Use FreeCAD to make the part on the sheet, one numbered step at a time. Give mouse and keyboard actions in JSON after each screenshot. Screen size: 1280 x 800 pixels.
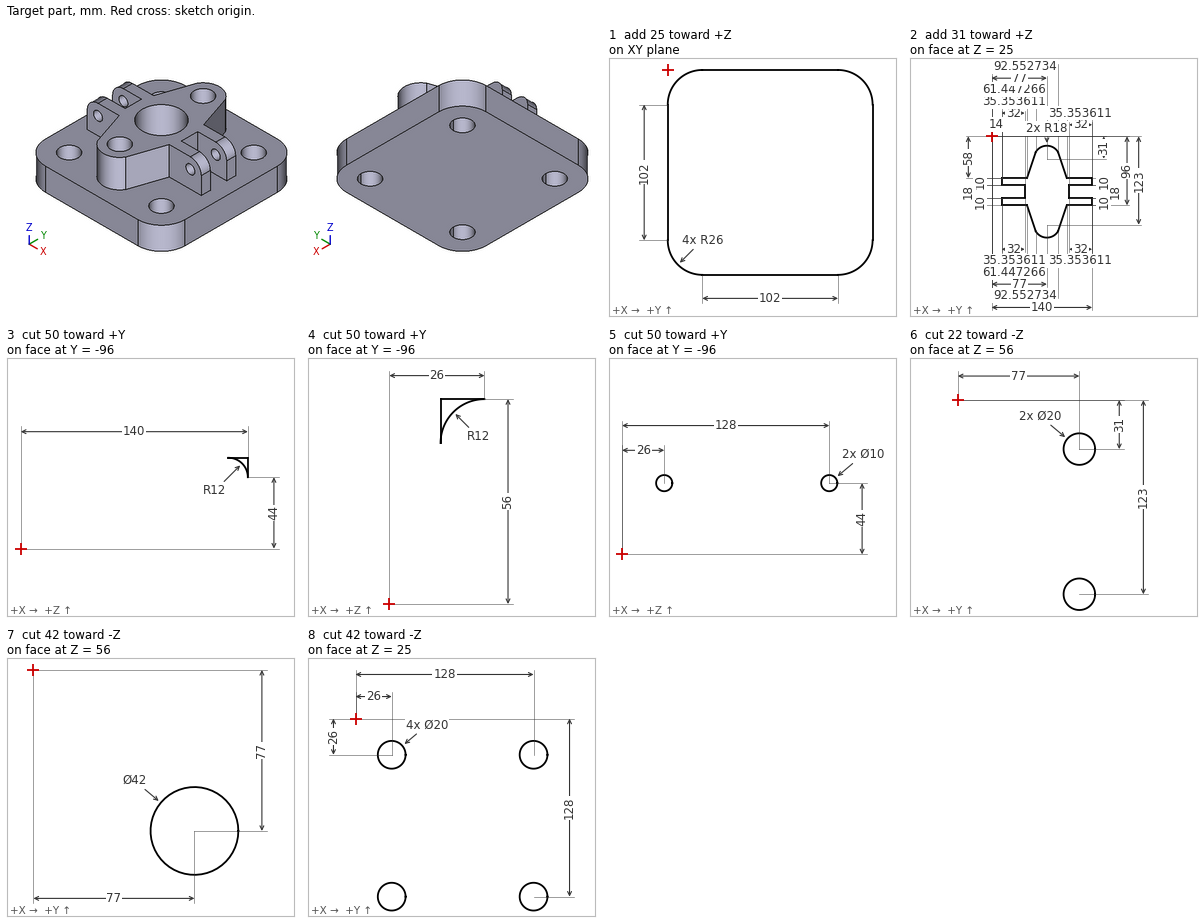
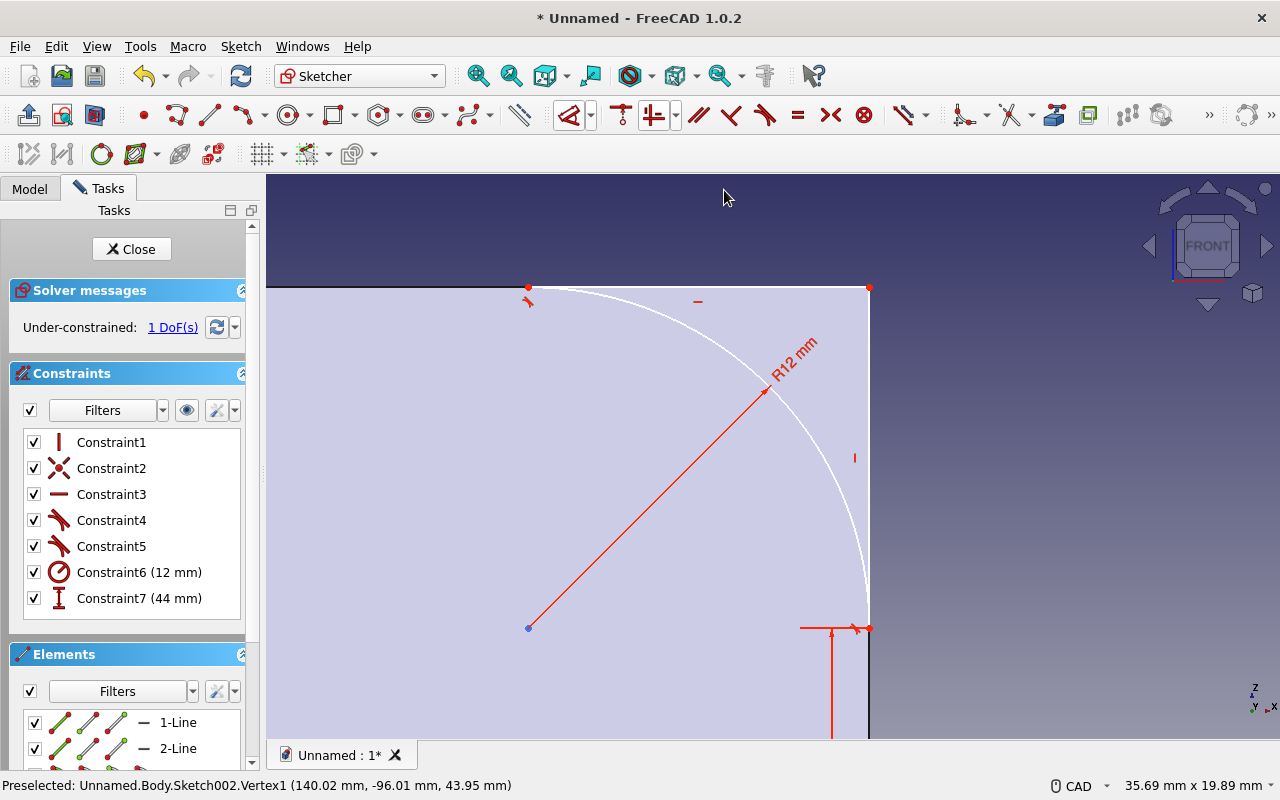
{"action": "left_click", "coordinate": [869, 628]}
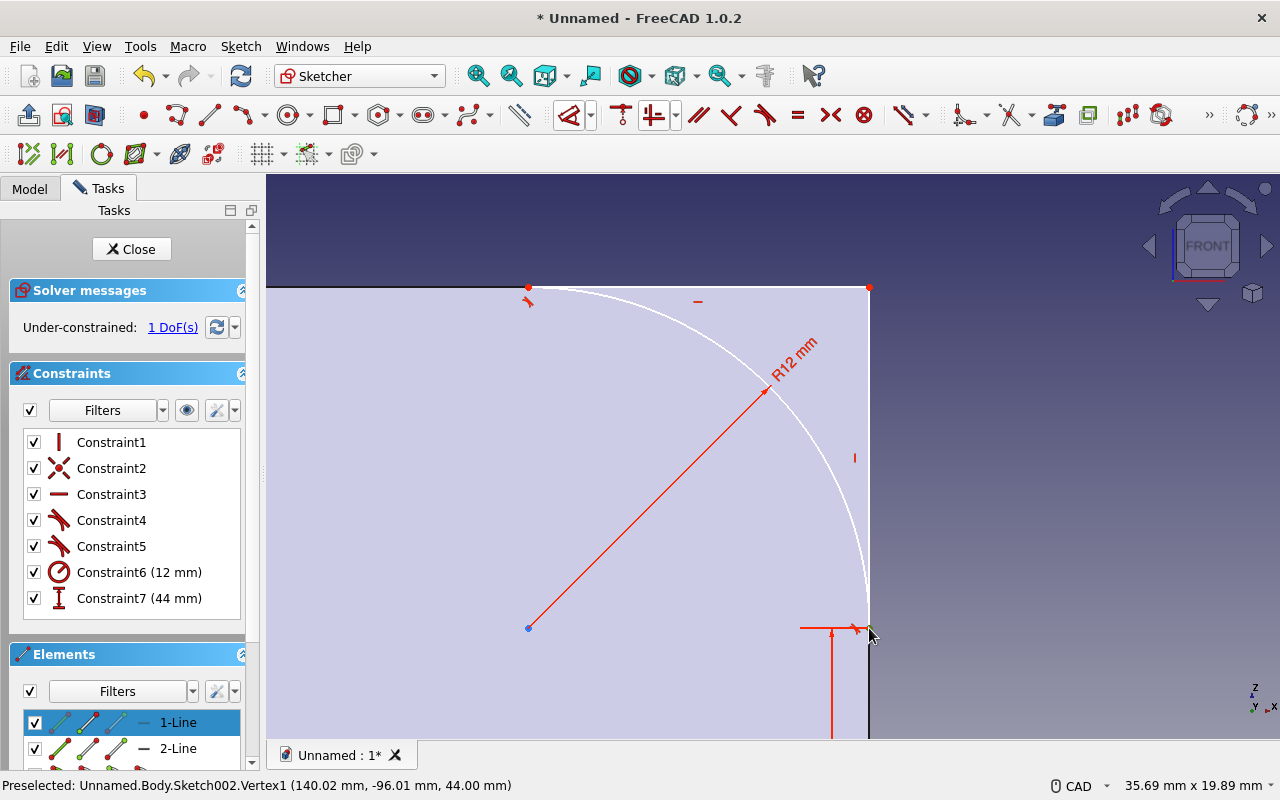
{"action": "key", "text": "l"}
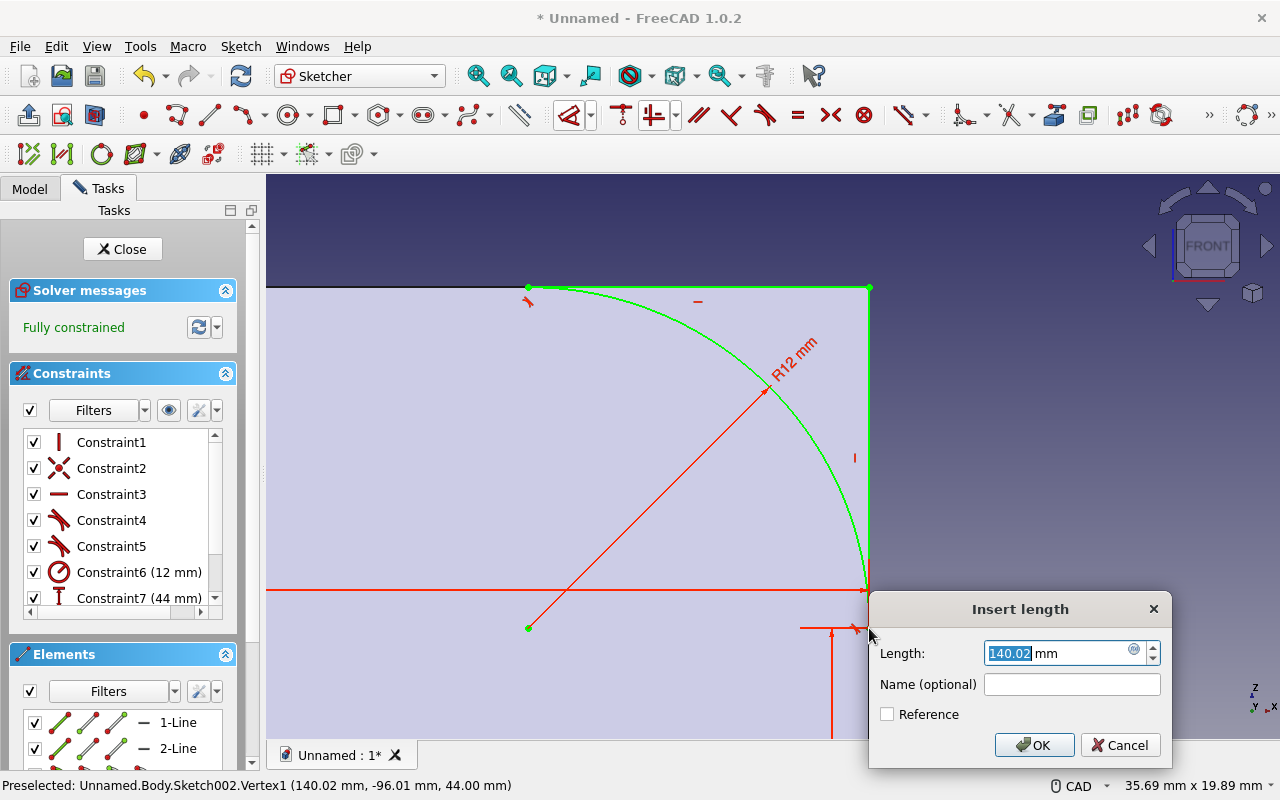
{"action": "type", "text": "140"}
{"action": "key", "text": "Return"}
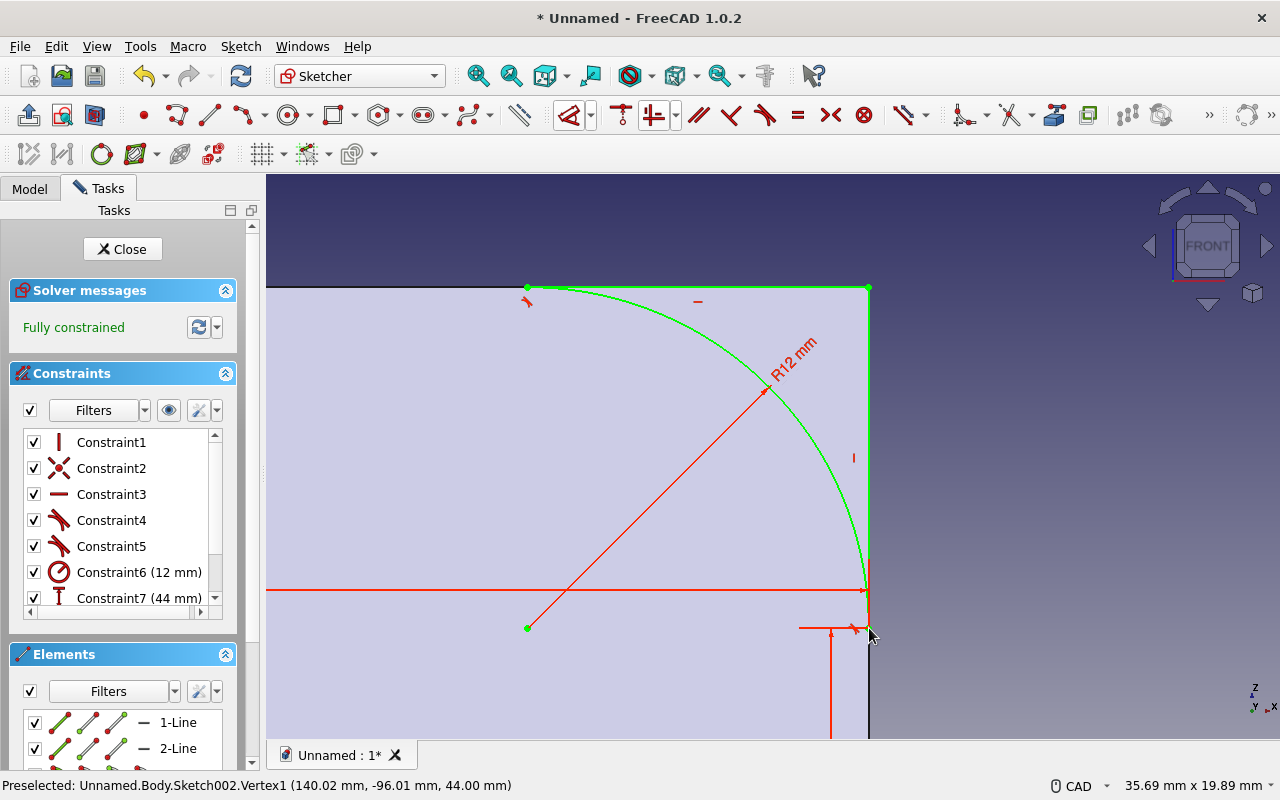
{"action": "left_click", "coordinate": [123, 249]}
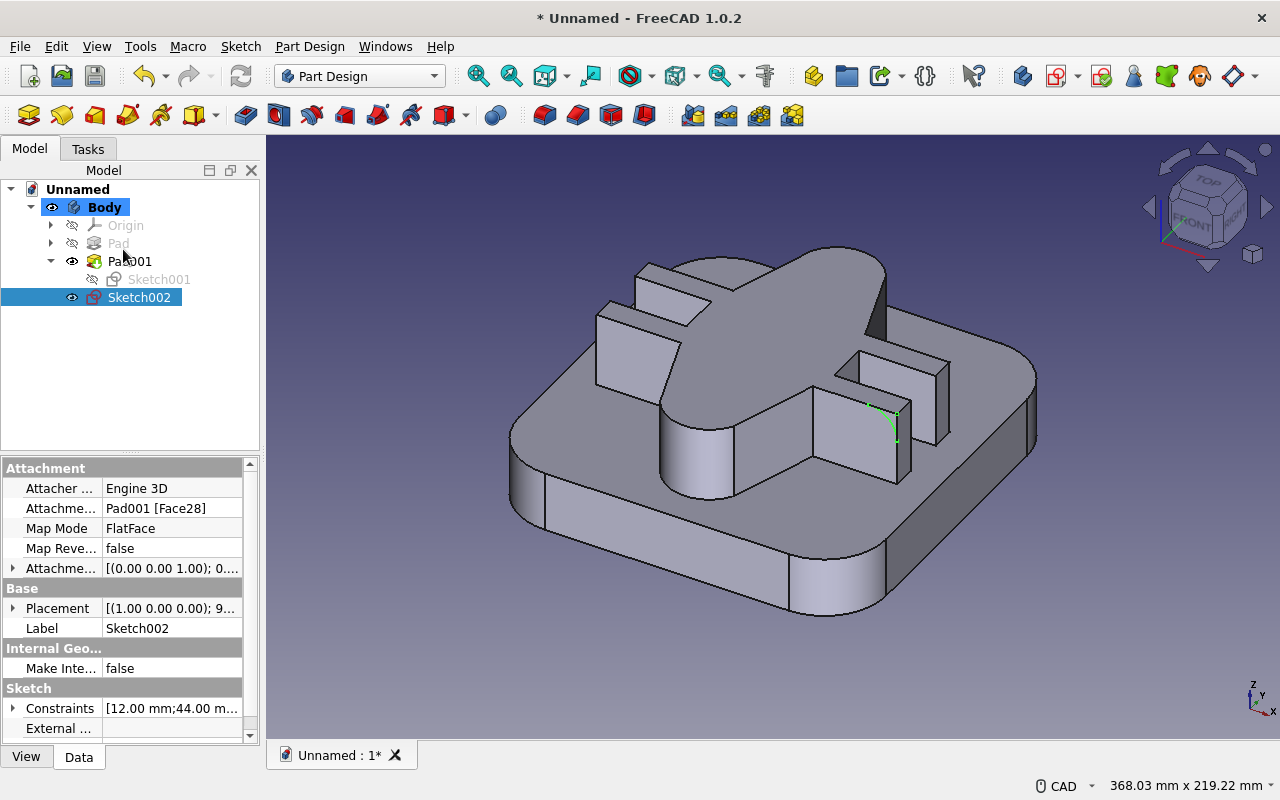
{"action": "left_click", "coordinate": [246, 116]}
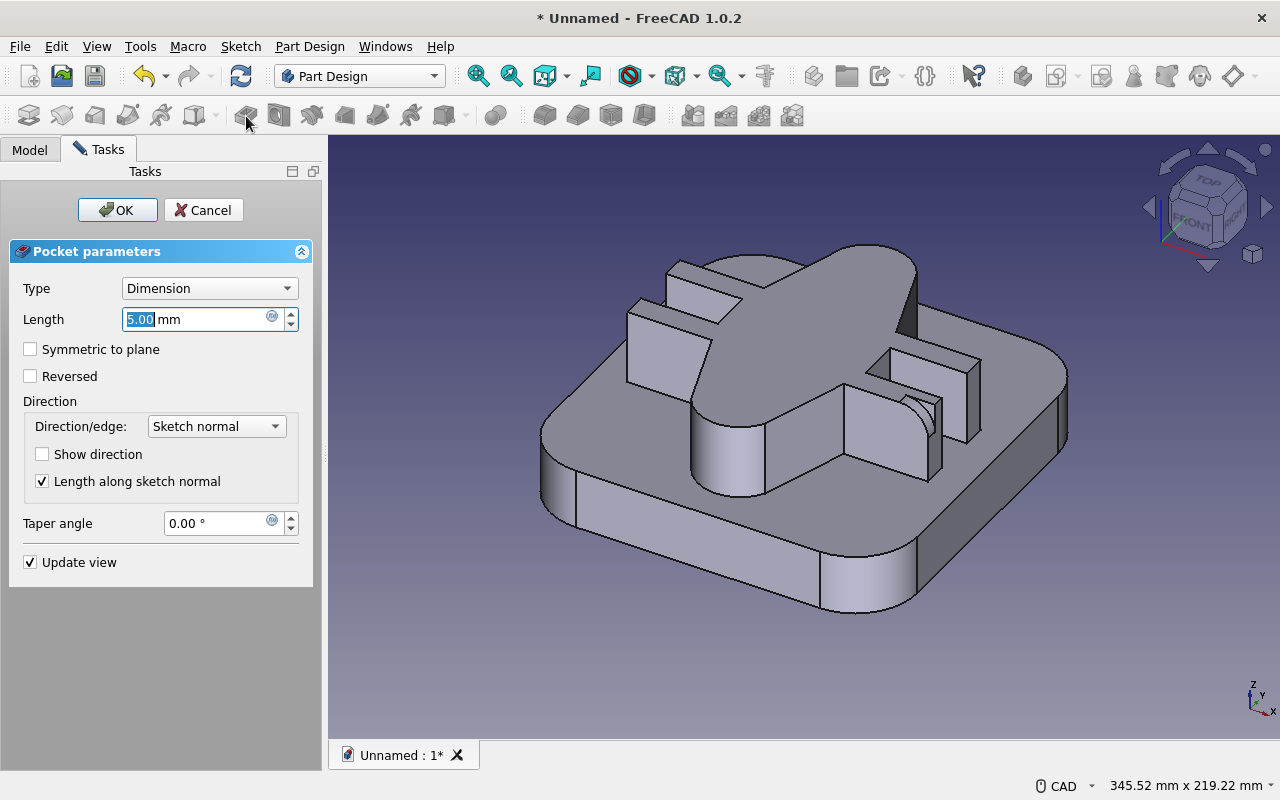
{"action": "type", "text": "50"}
{"action": "key", "text": "Tab"}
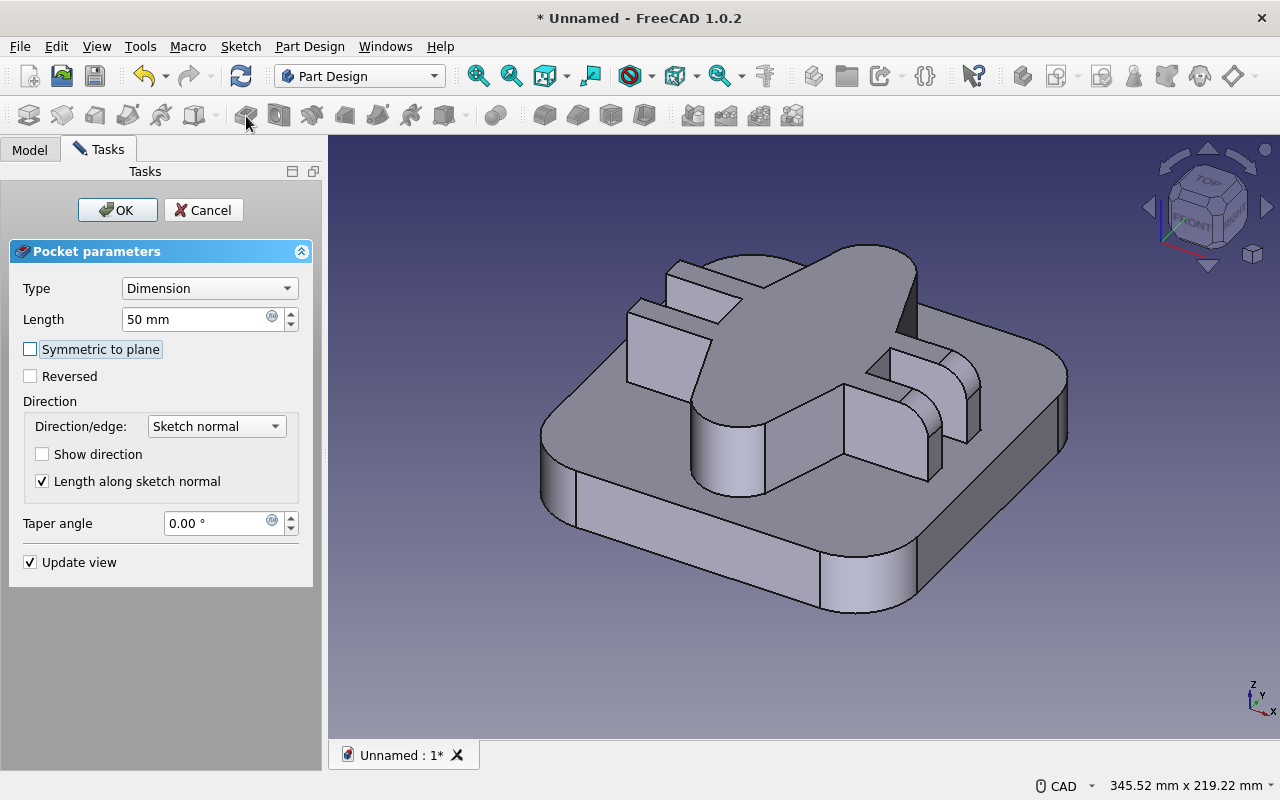
{"action": "left_click", "coordinate": [118, 210]}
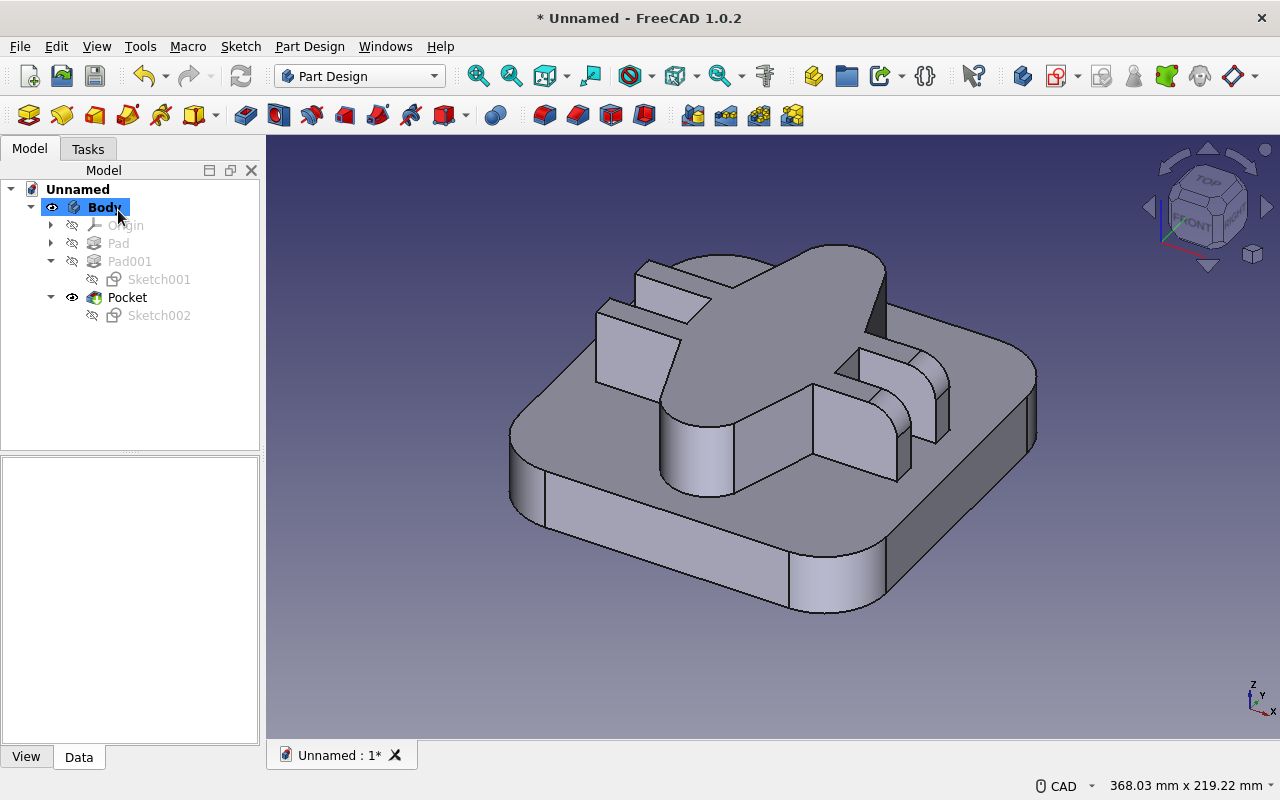
{"action": "left_click", "coordinate": [639, 360]}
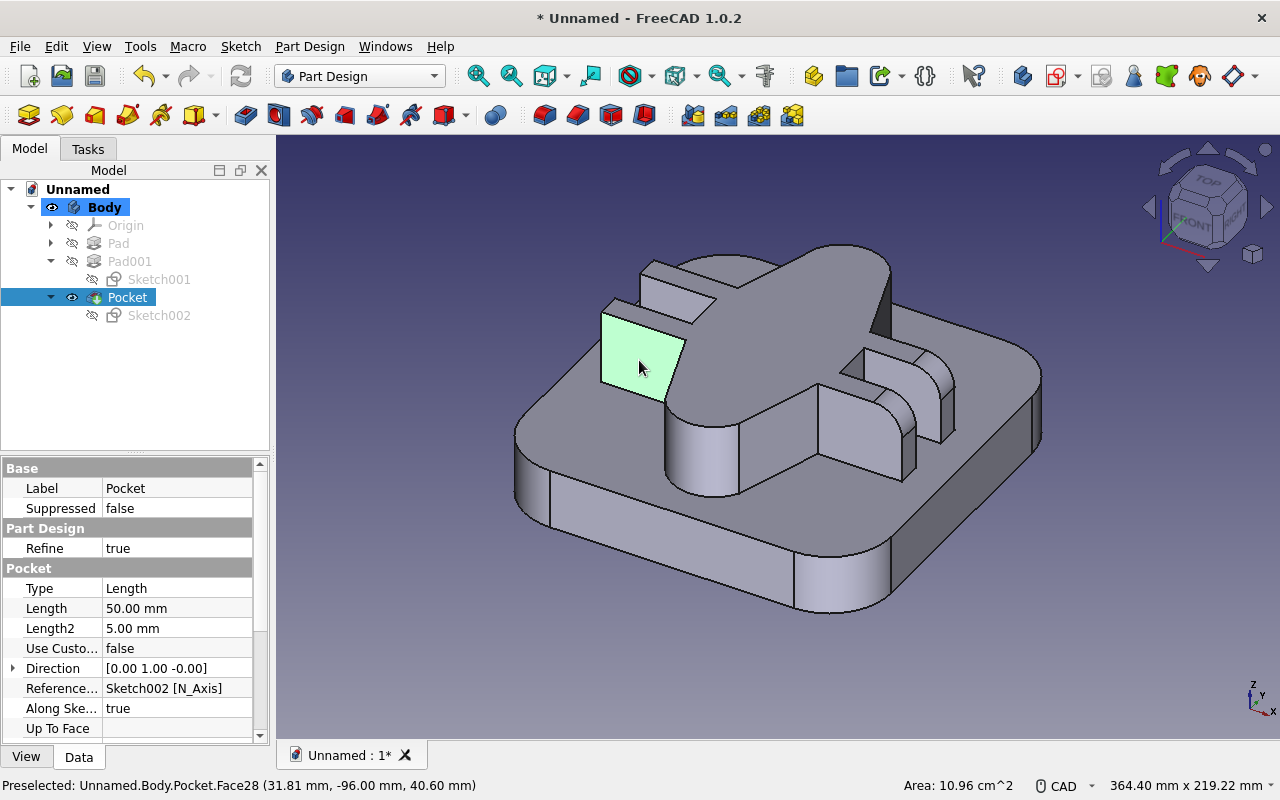
{"action": "left_click", "coordinate": [1056, 76]}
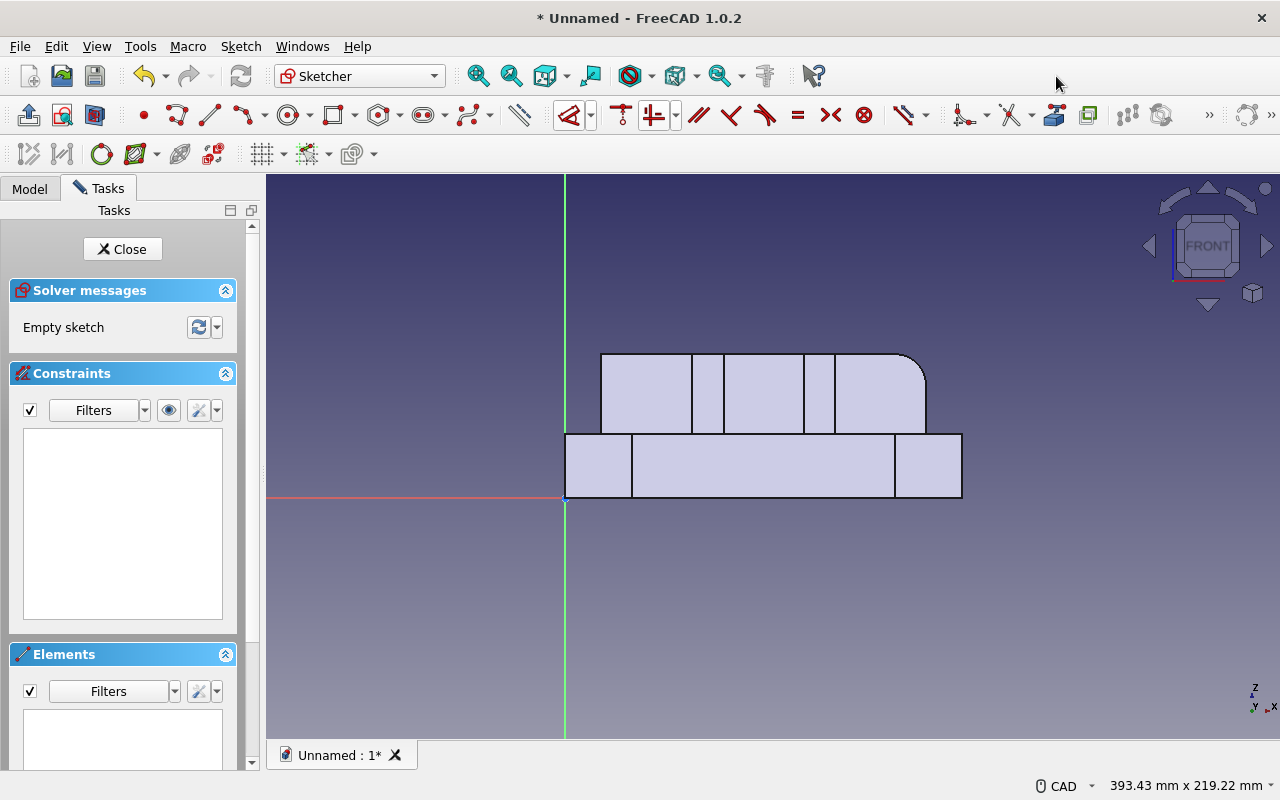
{"action": "scroll", "coordinate": [608, 361], "scroll_direction": "up", "scroll_amount": 12}